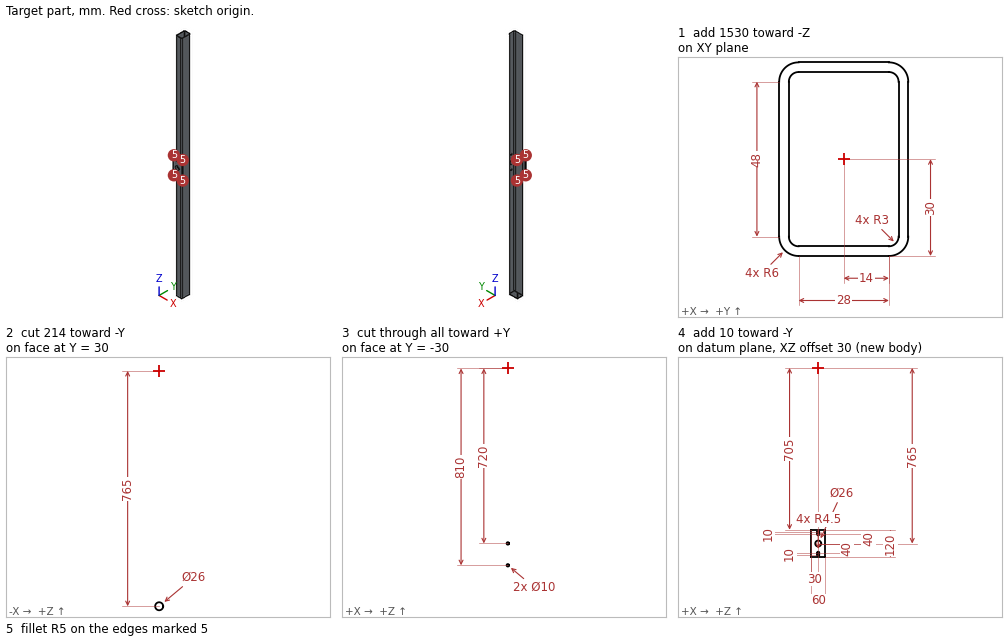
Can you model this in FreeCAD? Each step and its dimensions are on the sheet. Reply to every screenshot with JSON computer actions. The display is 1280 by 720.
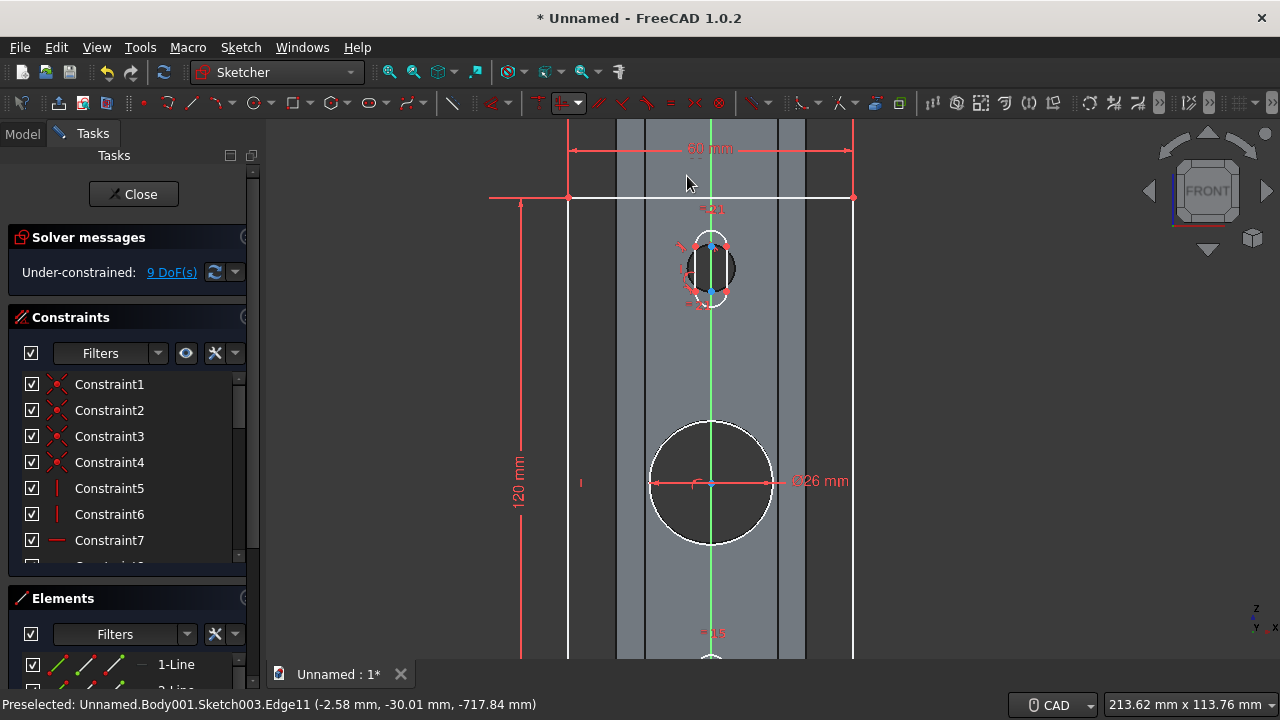
{"action": "scroll", "coordinate": [696, 276], "scroll_direction": "down", "scroll_amount": 3}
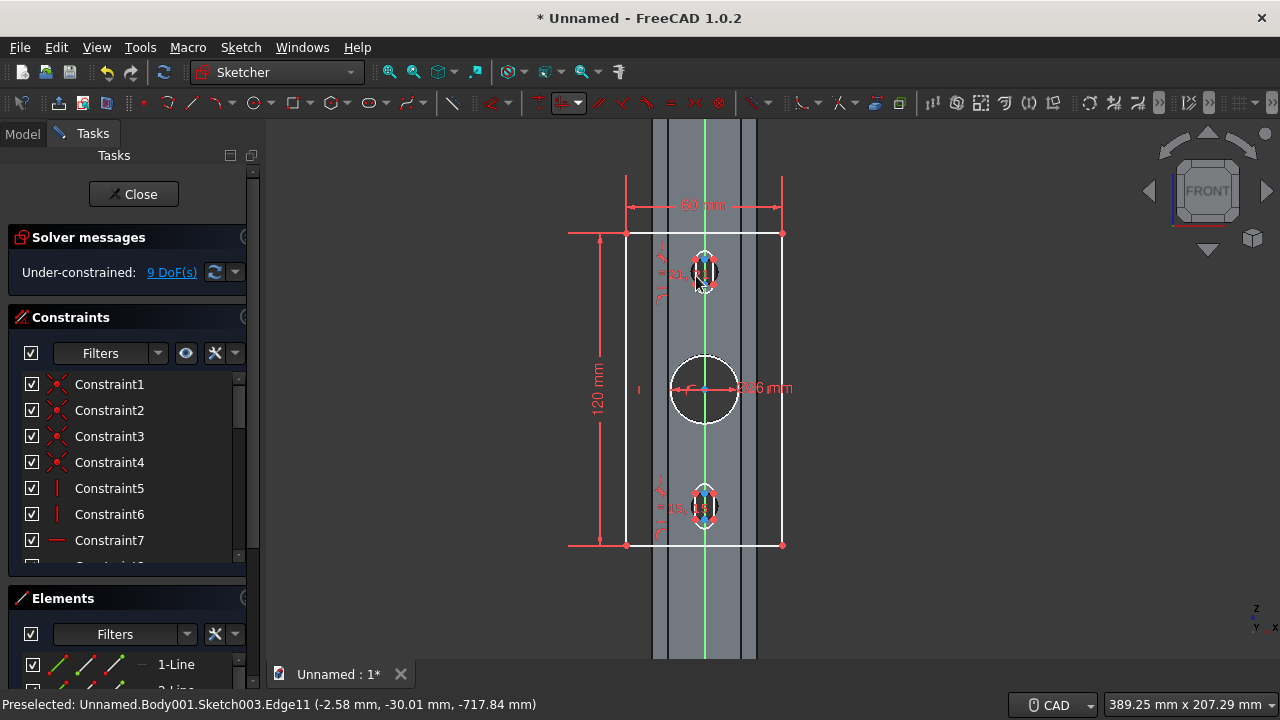
{"action": "scroll", "coordinate": [699, 527], "scroll_direction": "up", "scroll_amount": 5}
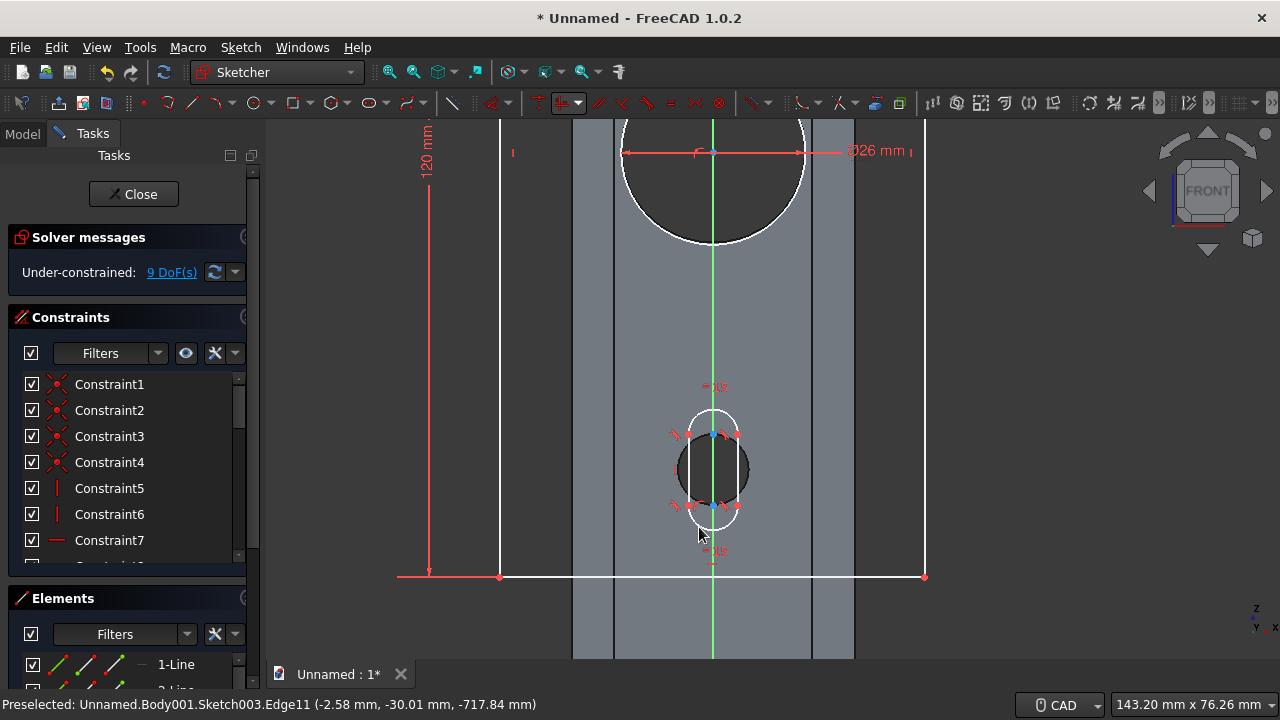
{"action": "left_click", "coordinate": [699, 526]}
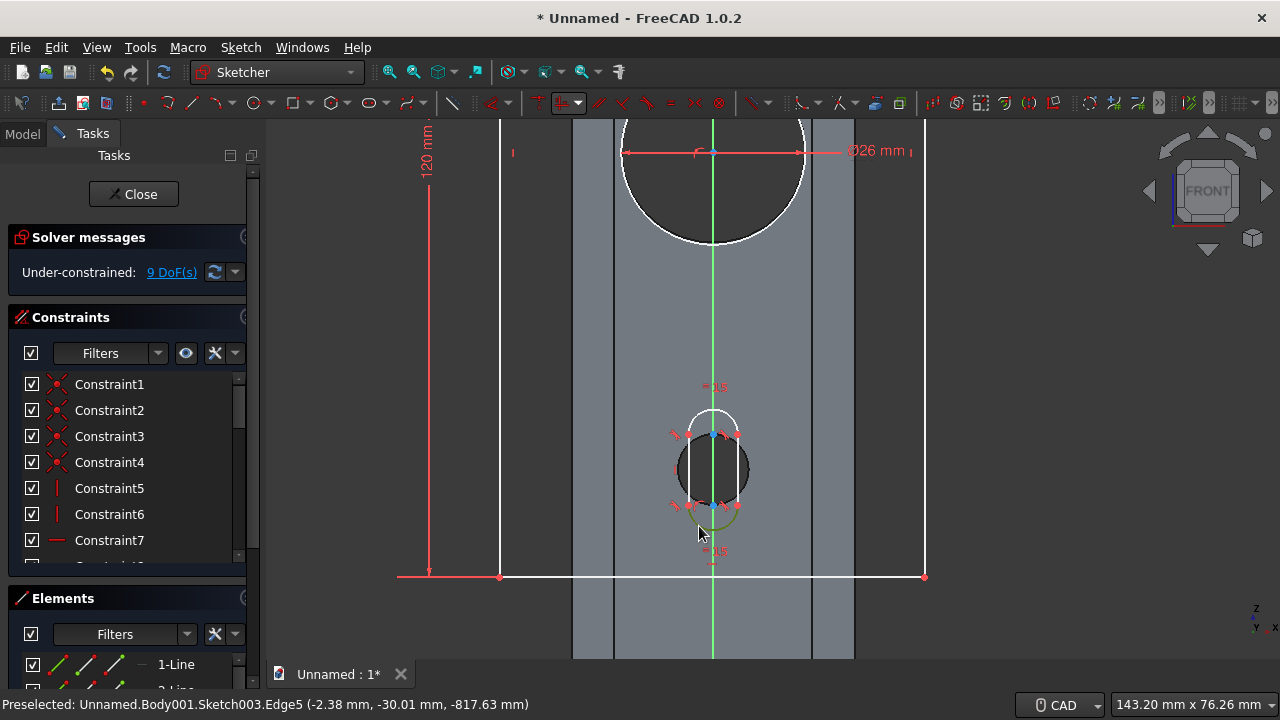
{"action": "scroll", "coordinate": [699, 528], "scroll_direction": "down", "scroll_amount": 5}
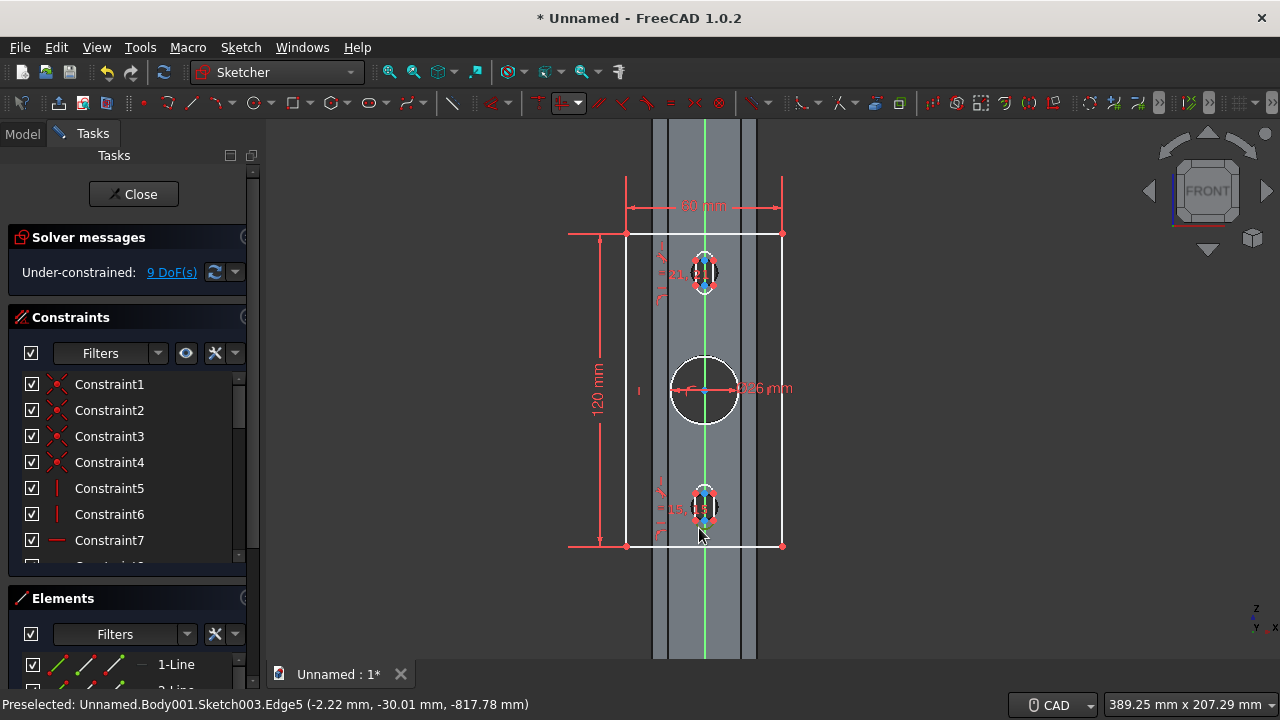
{"action": "scroll", "coordinate": [699, 292], "scroll_direction": "up", "scroll_amount": 5}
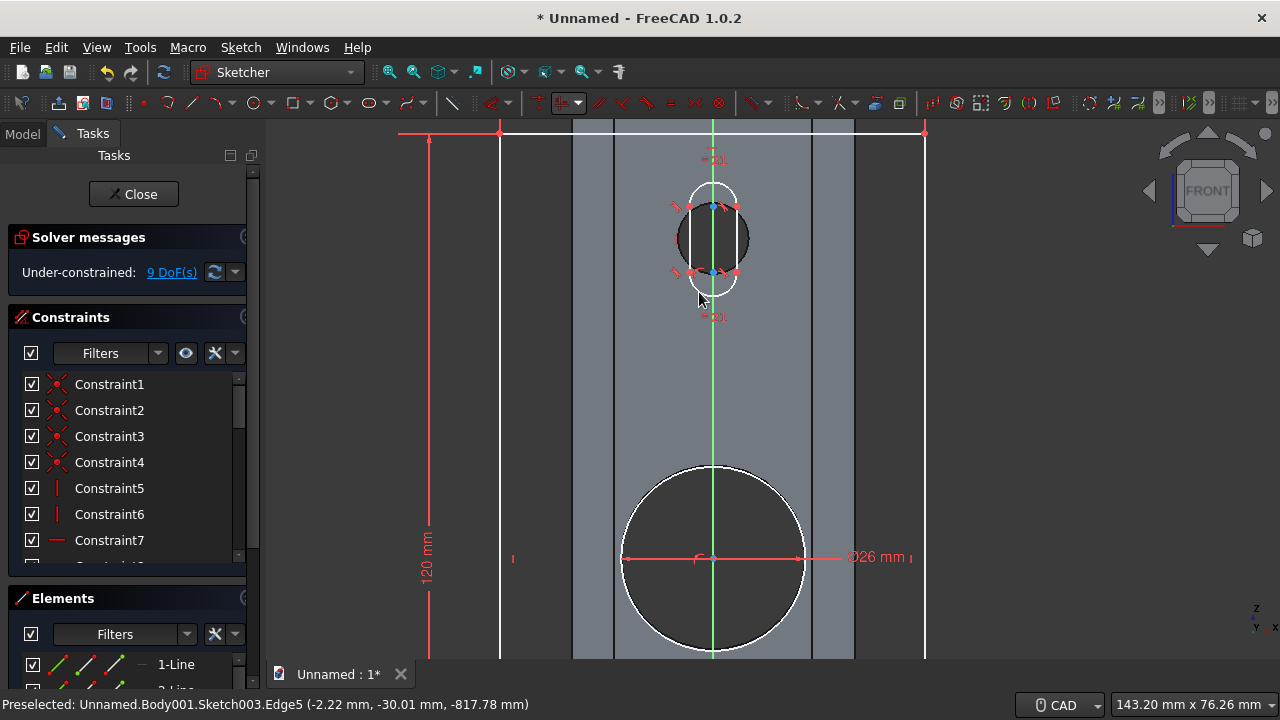
{"action": "left_click", "coordinate": [699, 292]}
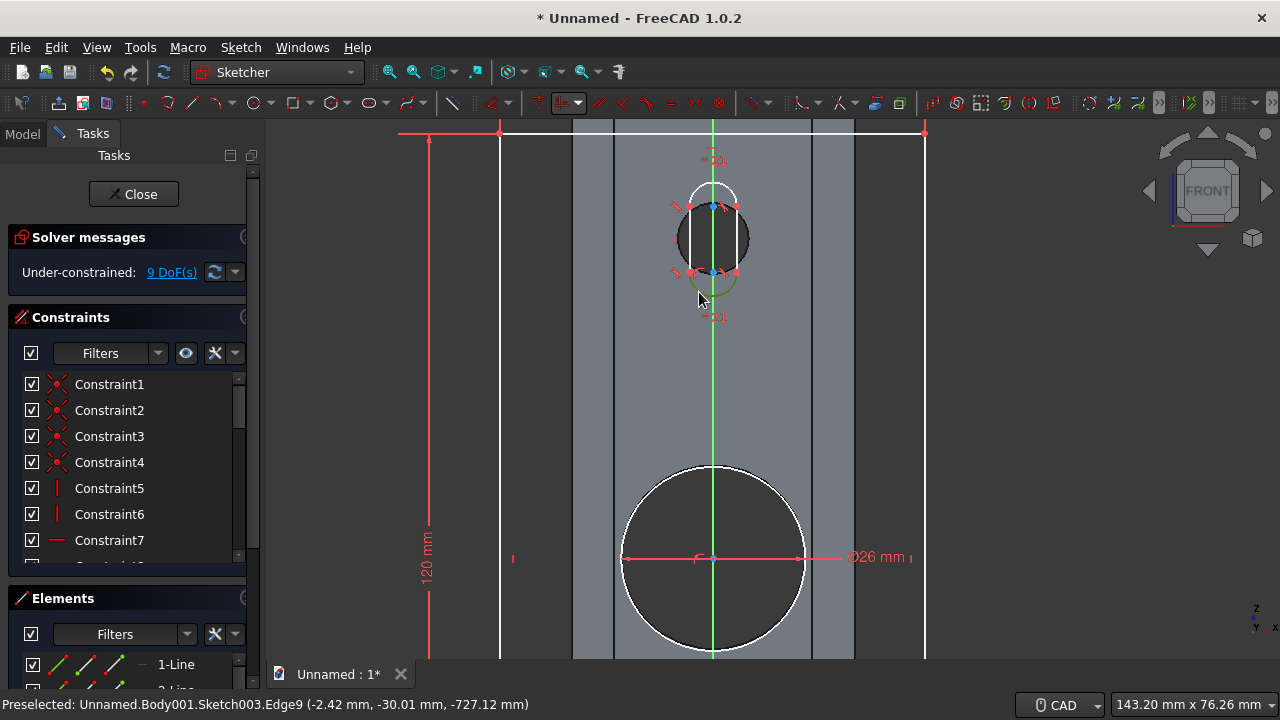
{"action": "left_click", "coordinate": [672, 104]}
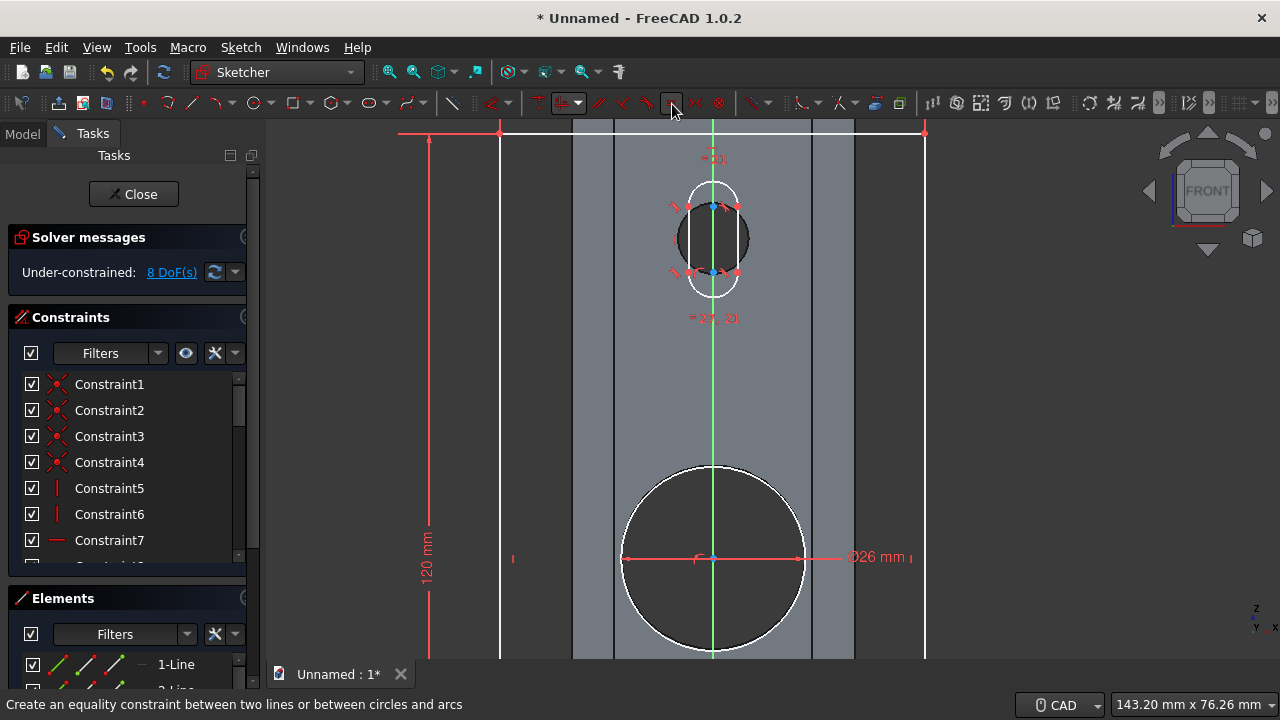
{"action": "left_click", "coordinate": [492, 104]}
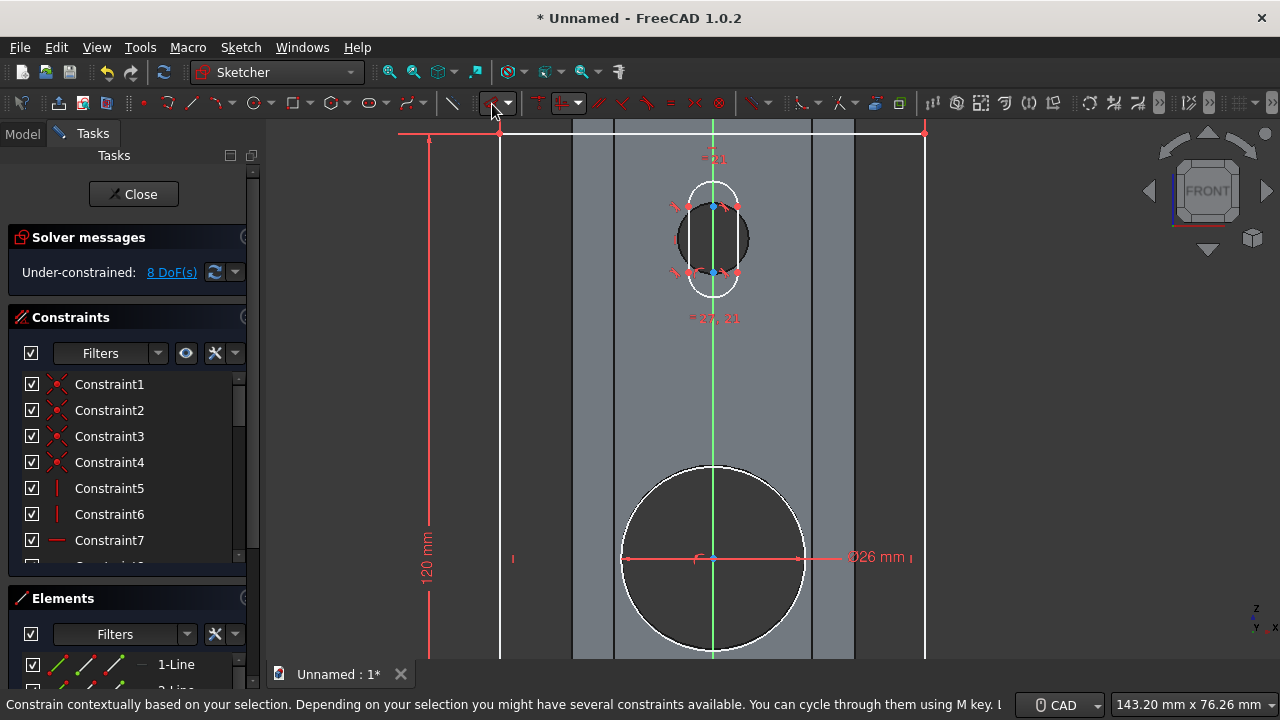
{"action": "scroll", "coordinate": [699, 291], "scroll_direction": "down", "scroll_amount": 5}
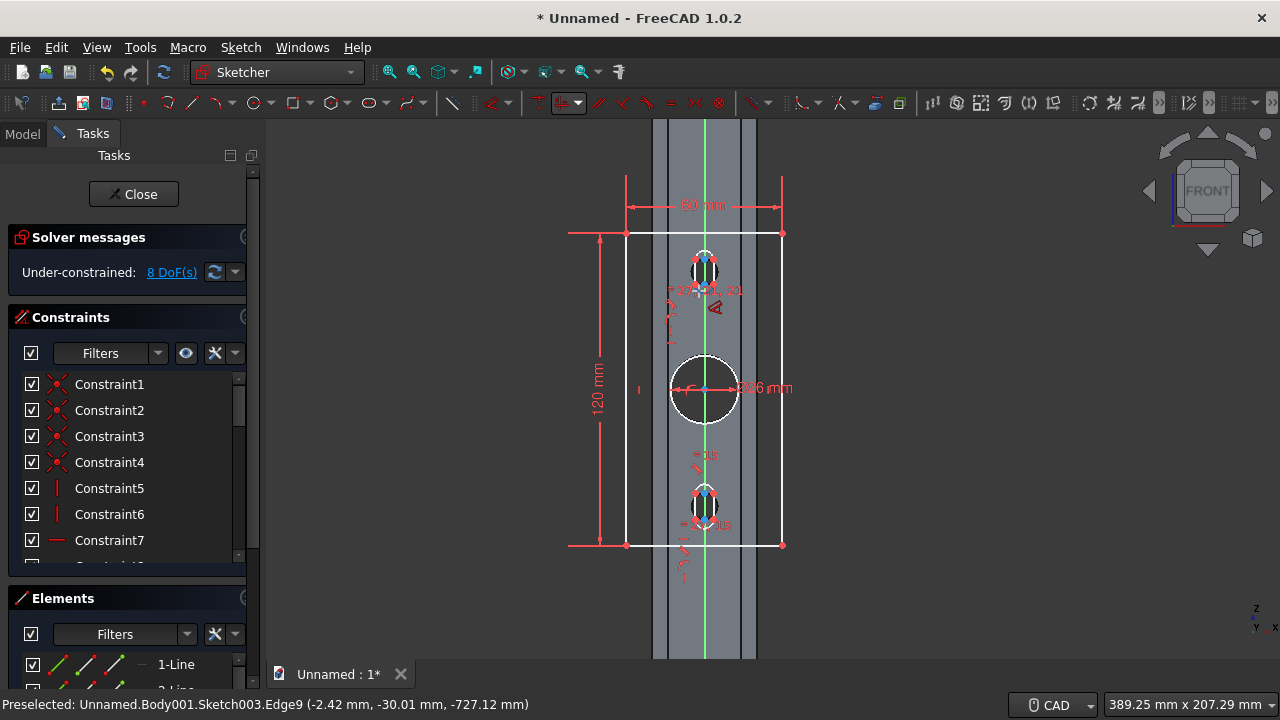
{"action": "scroll", "coordinate": [699, 527], "scroll_direction": "up", "scroll_amount": 7}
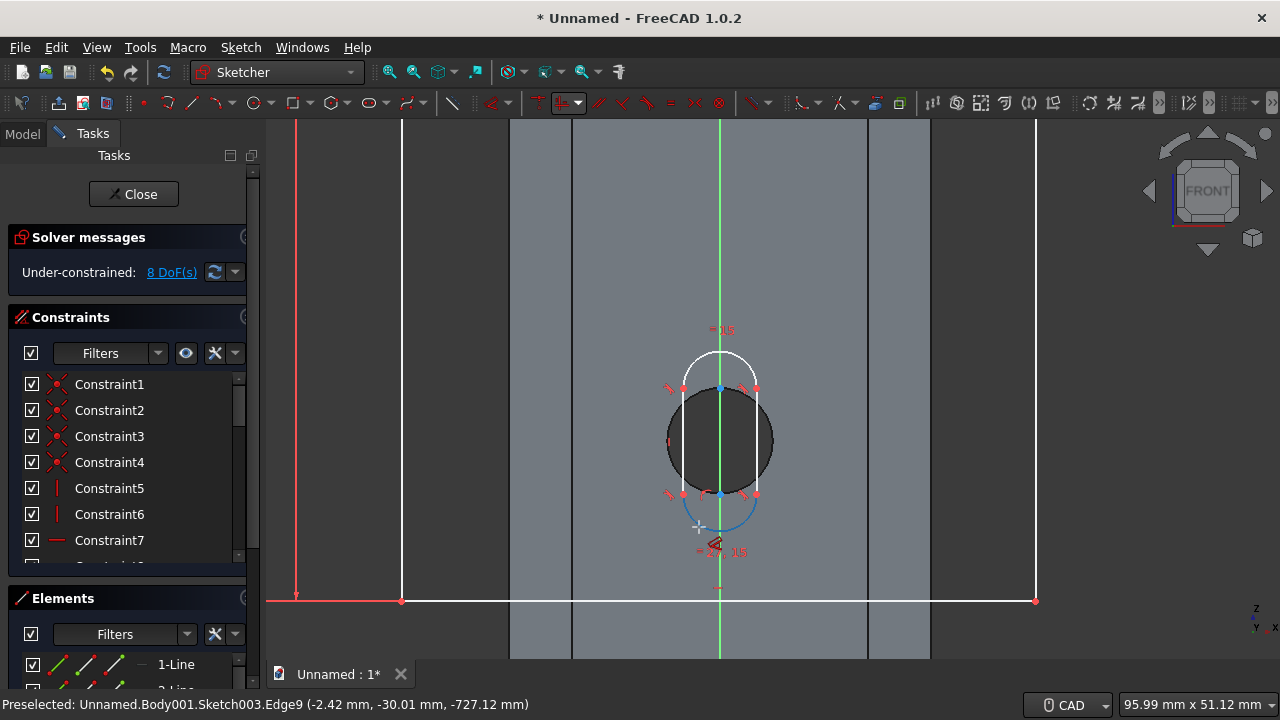
{"action": "left_click", "coordinate": [699, 524]}
{"action": "left_click", "coordinate": [680, 550]}